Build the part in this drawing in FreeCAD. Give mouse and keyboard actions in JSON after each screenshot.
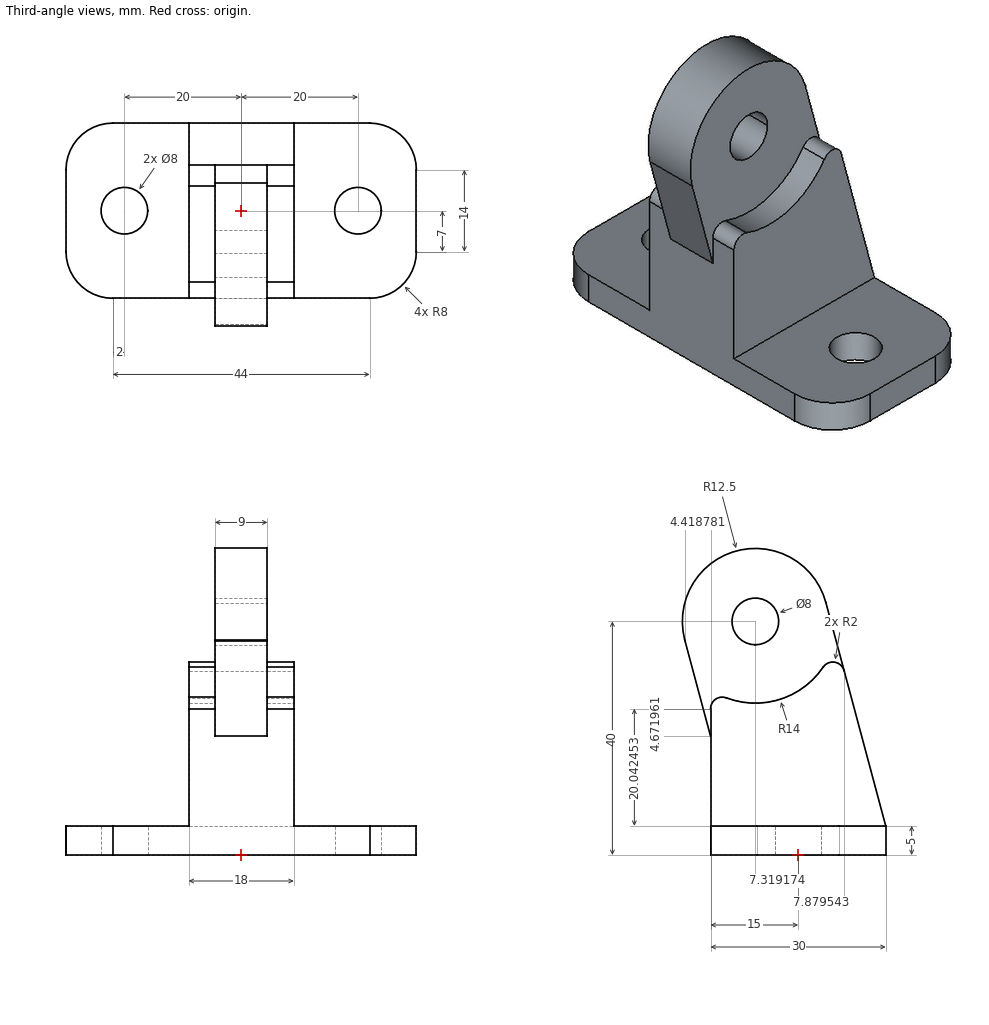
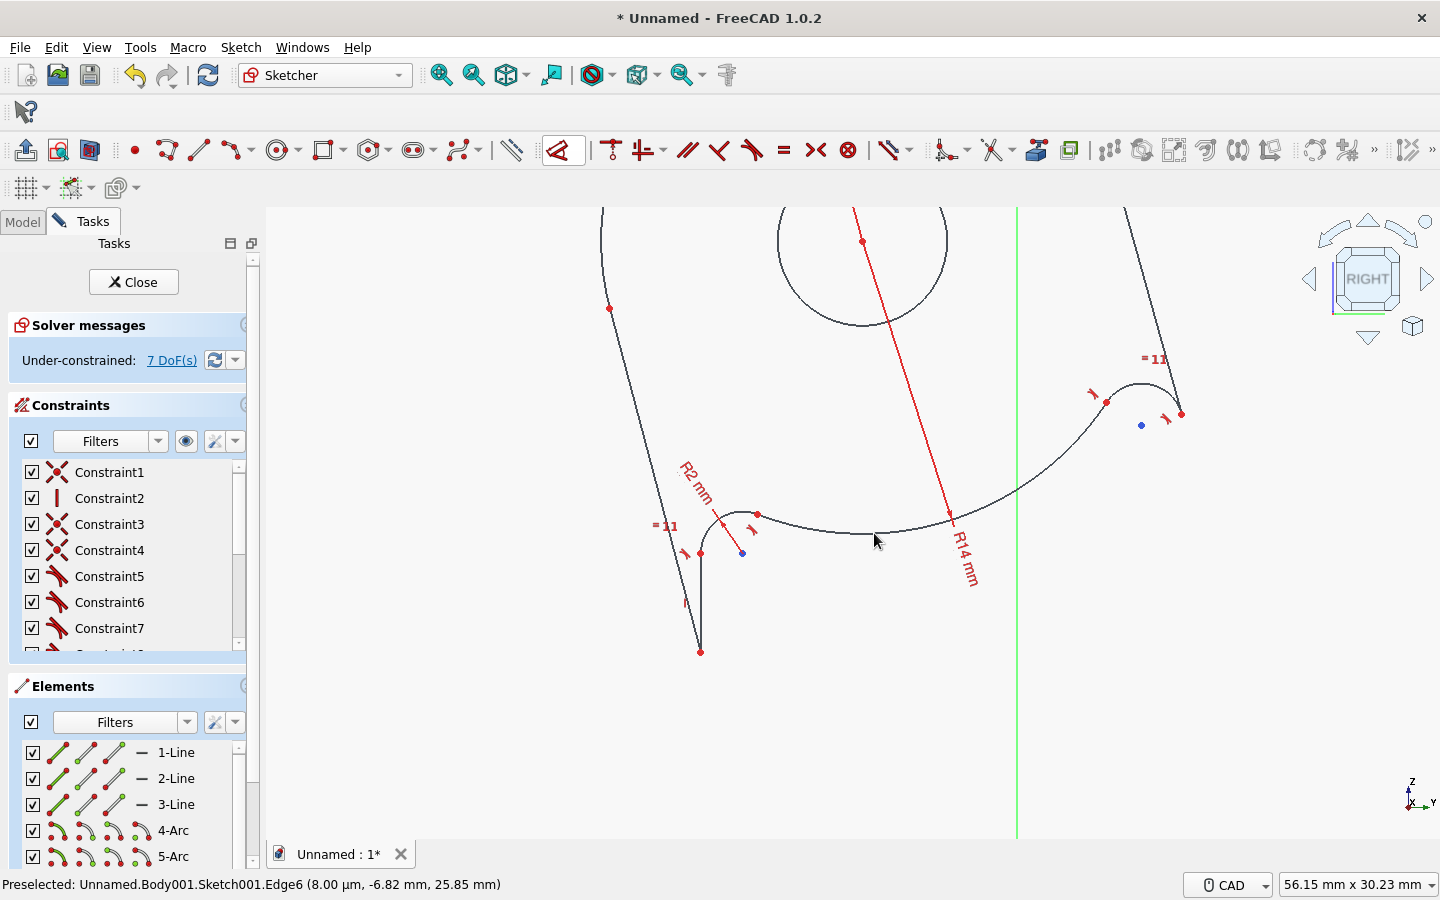
{"action": "left_click", "coordinate": [803, 301]}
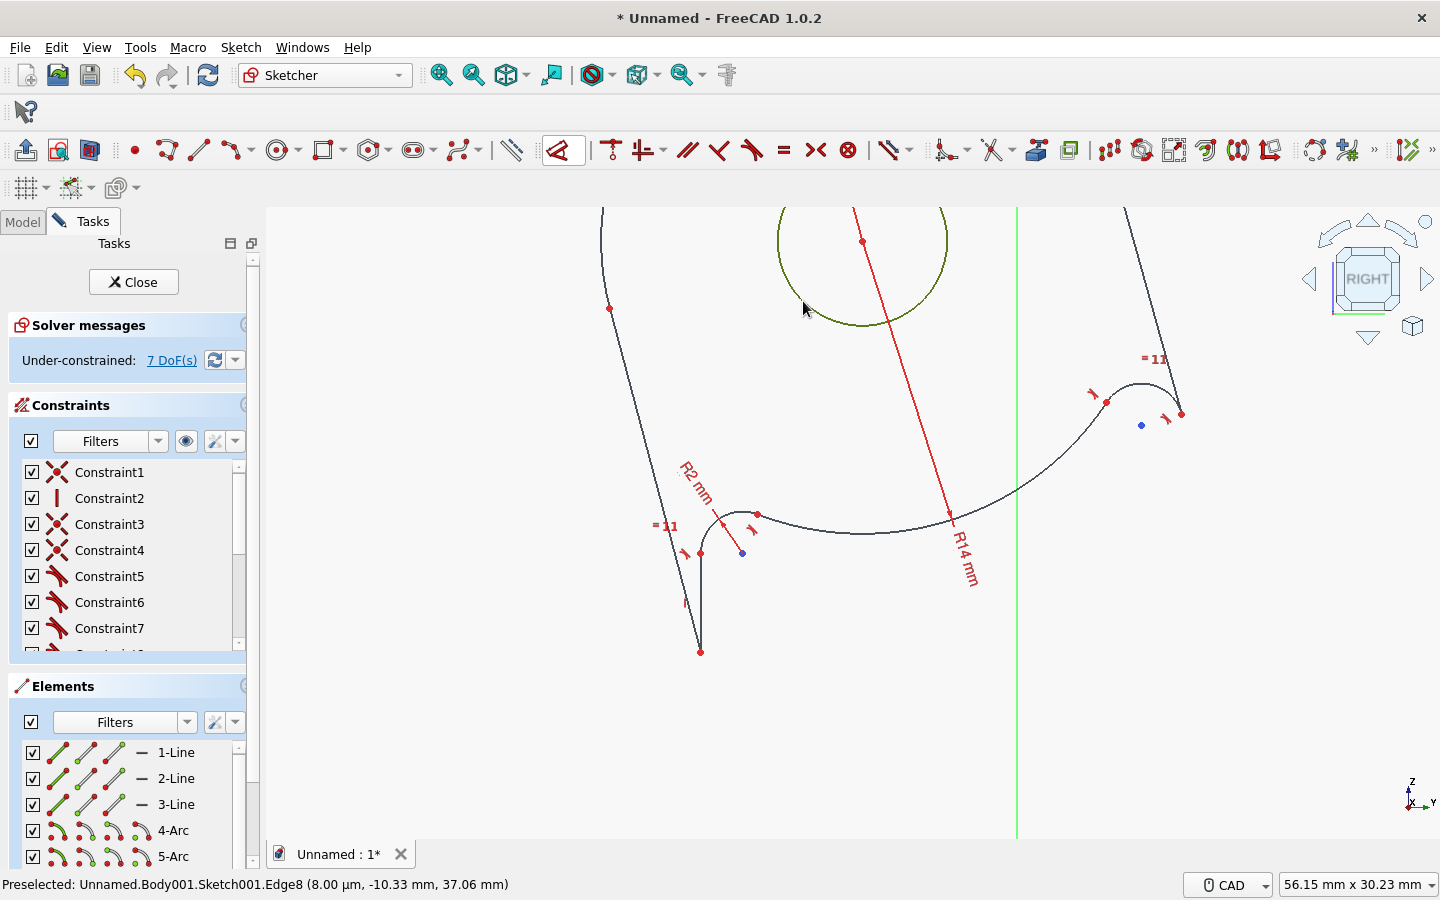
{"action": "key", "text": "k o"}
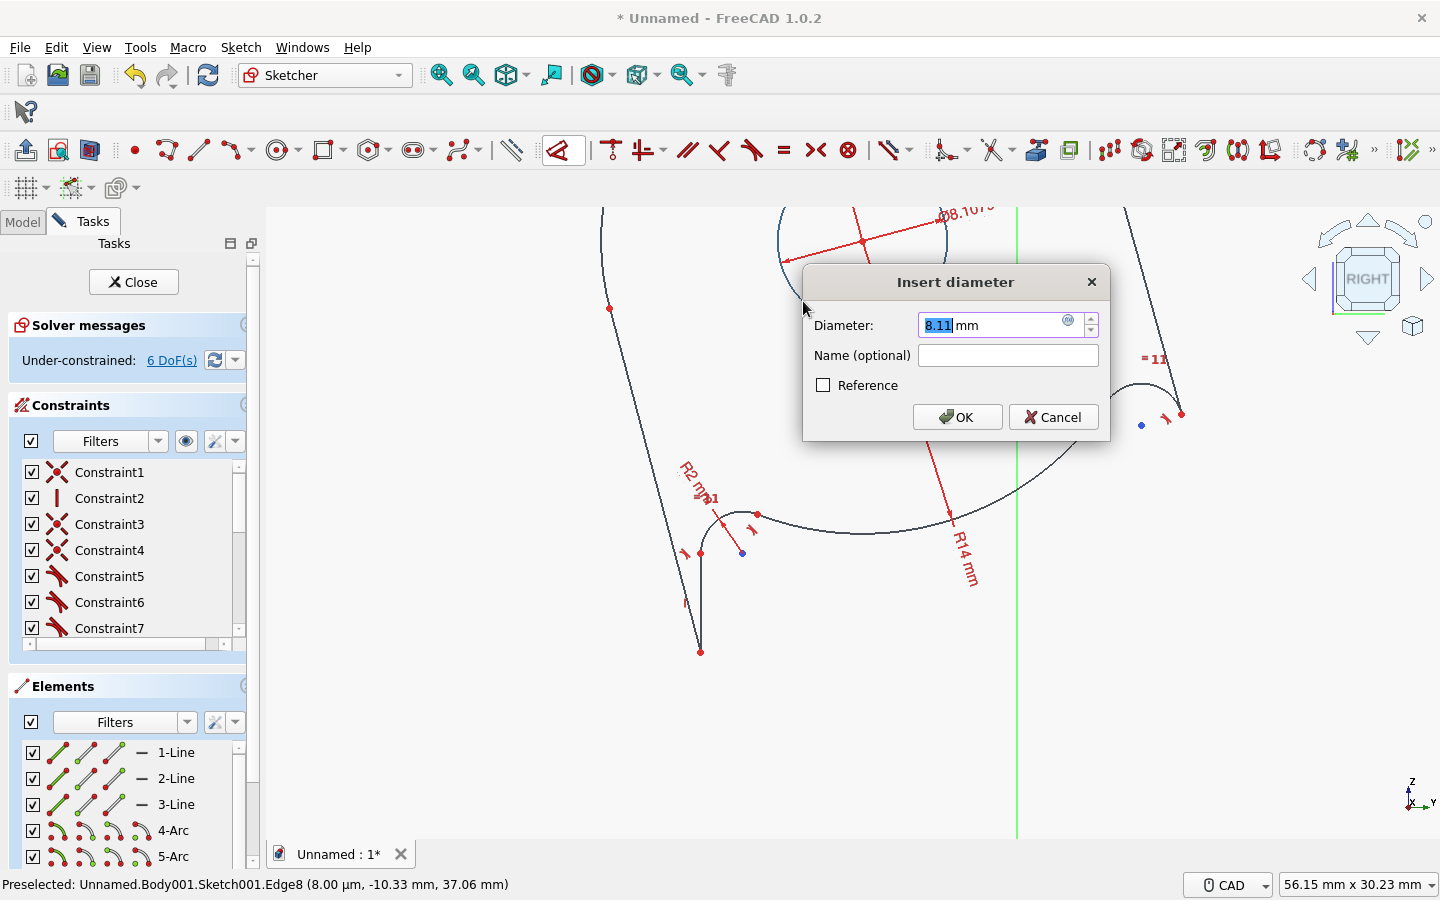
{"action": "type", "text": "8"}
{"action": "key", "text": "Return"}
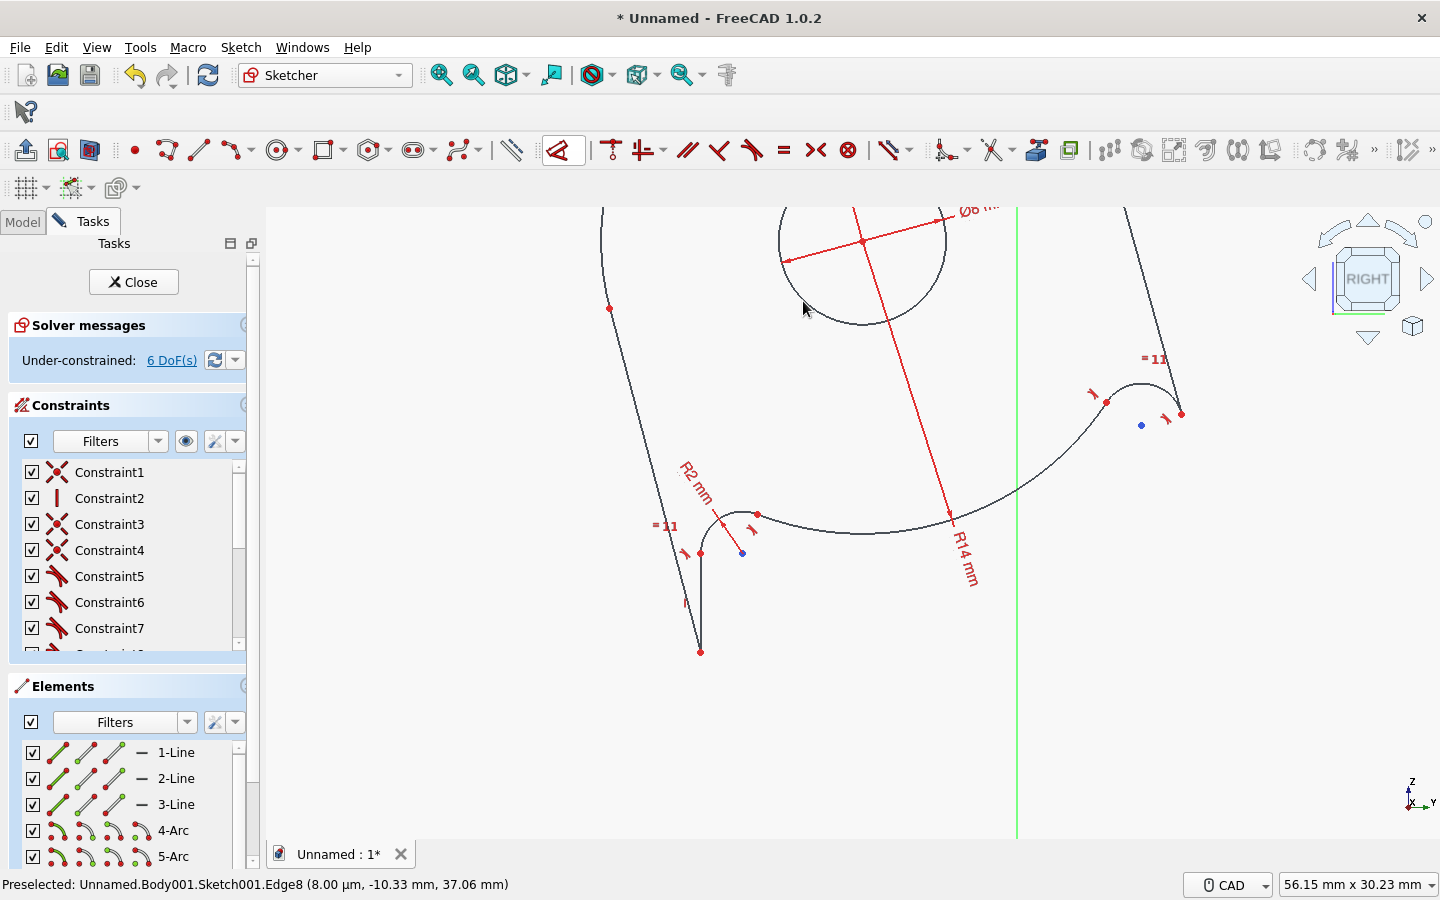
{"action": "left_click", "coordinate": [862, 241]}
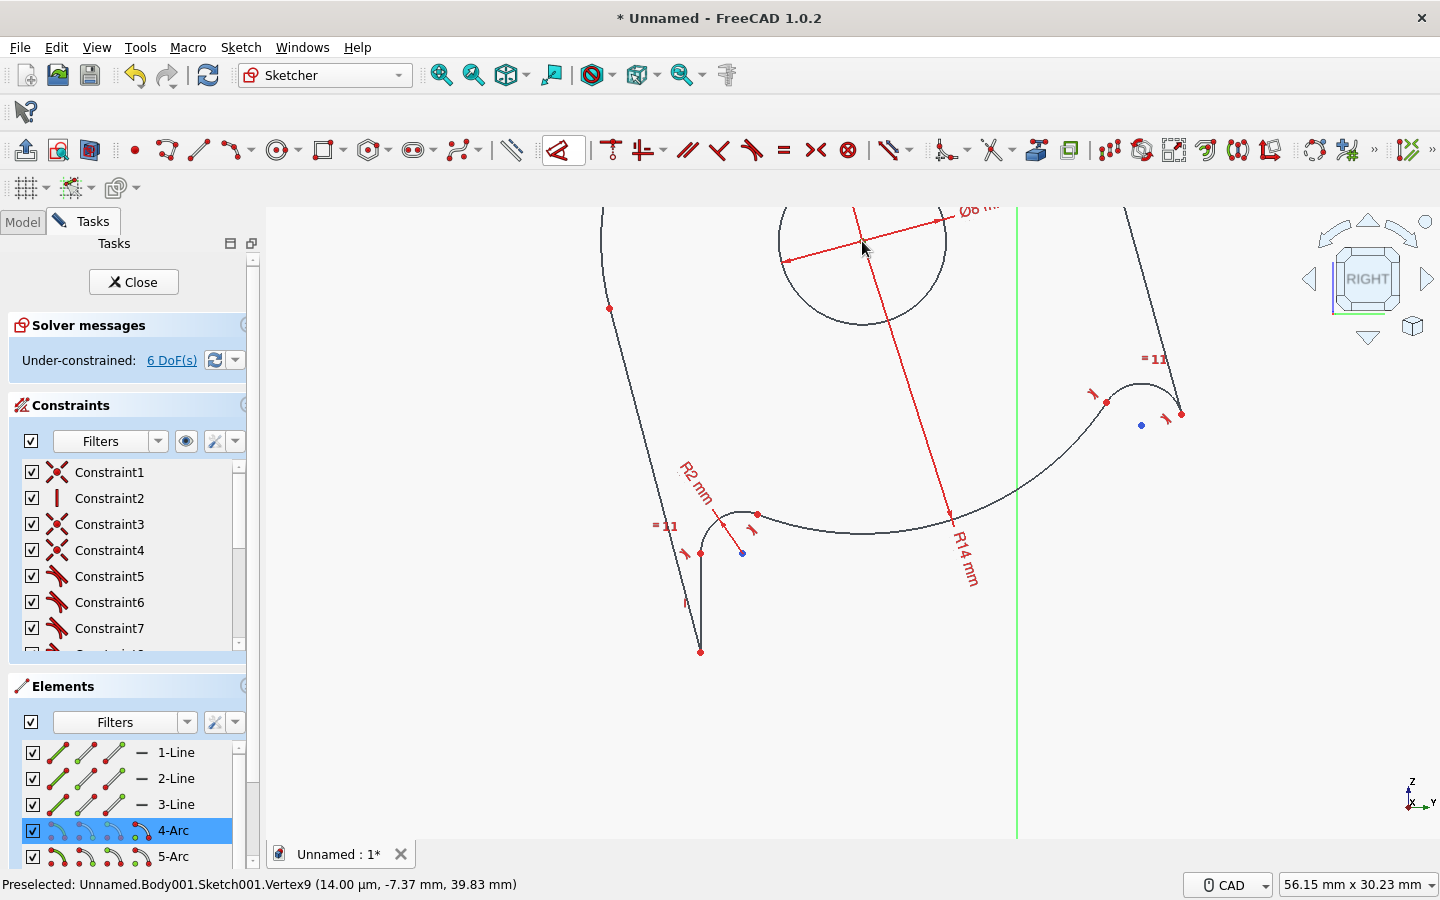
{"action": "key", "text": "i"}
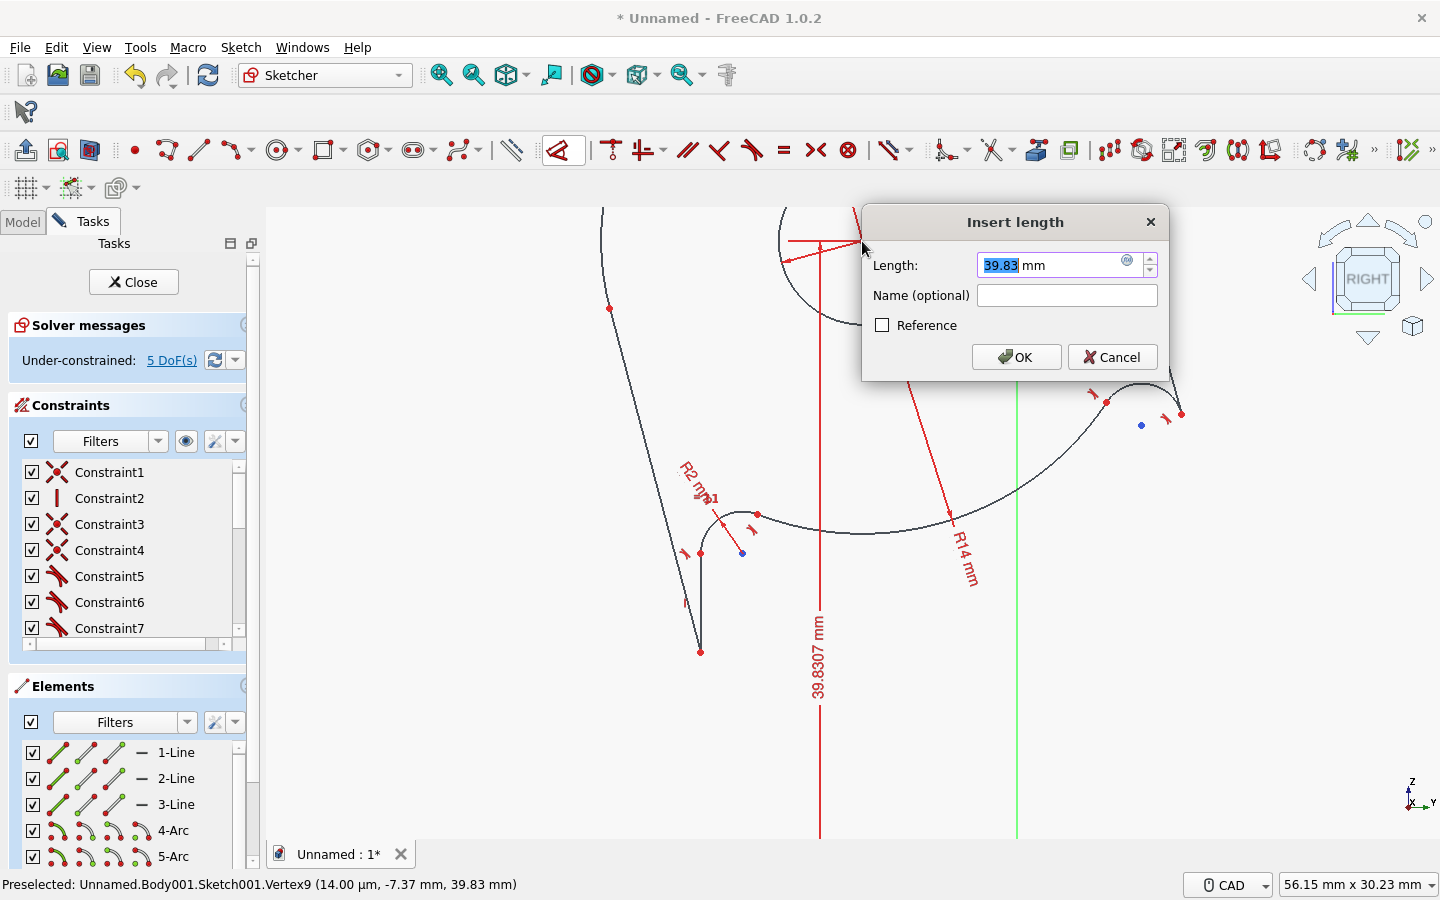
{"action": "type", "text": "40"}
{"action": "key", "text": "Return"}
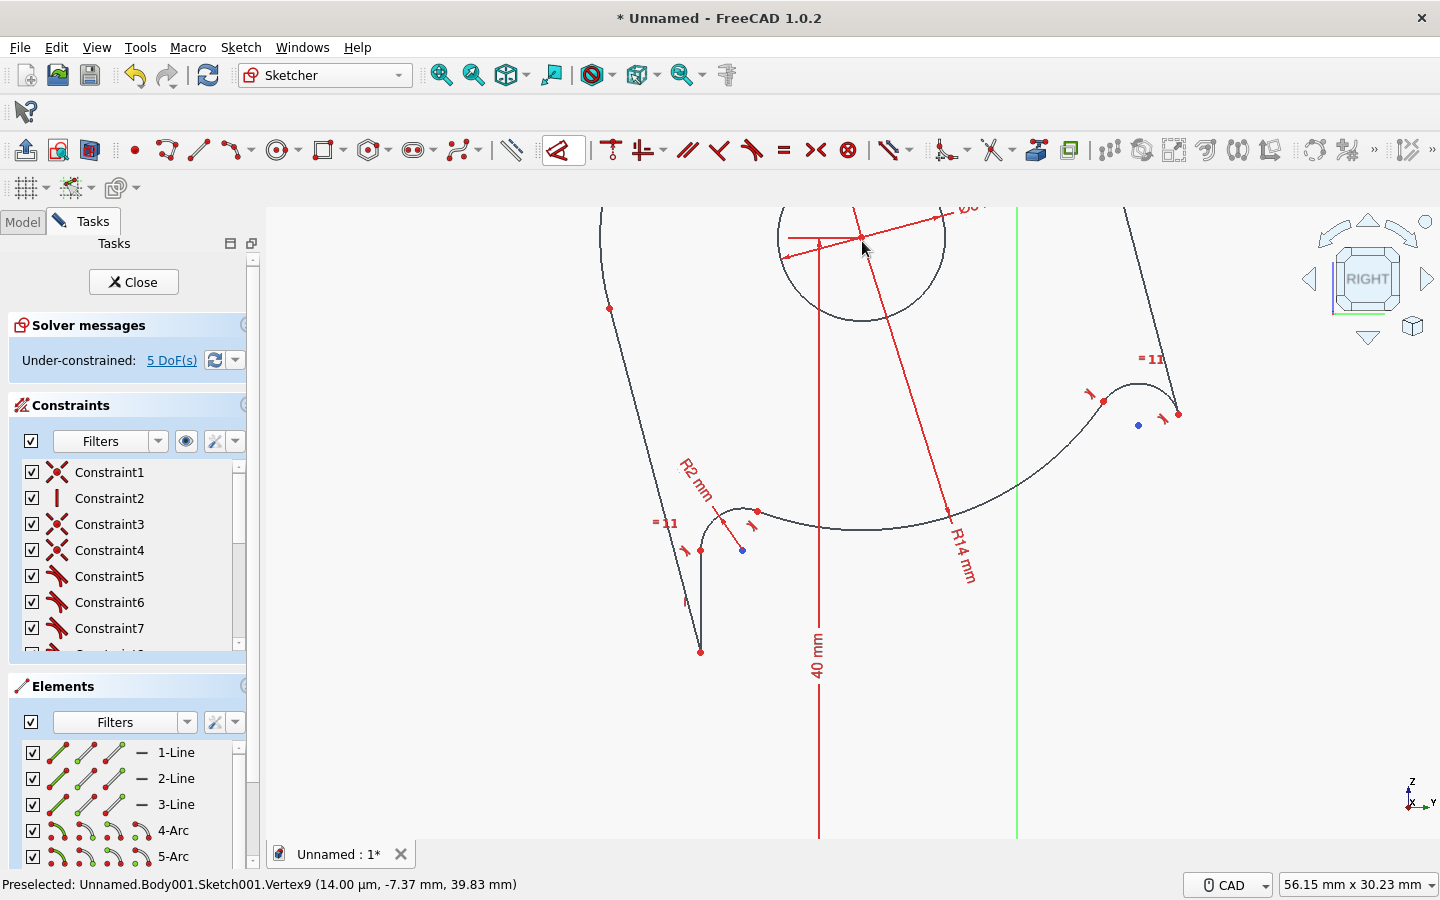
{"action": "left_click", "coordinate": [701, 652]}